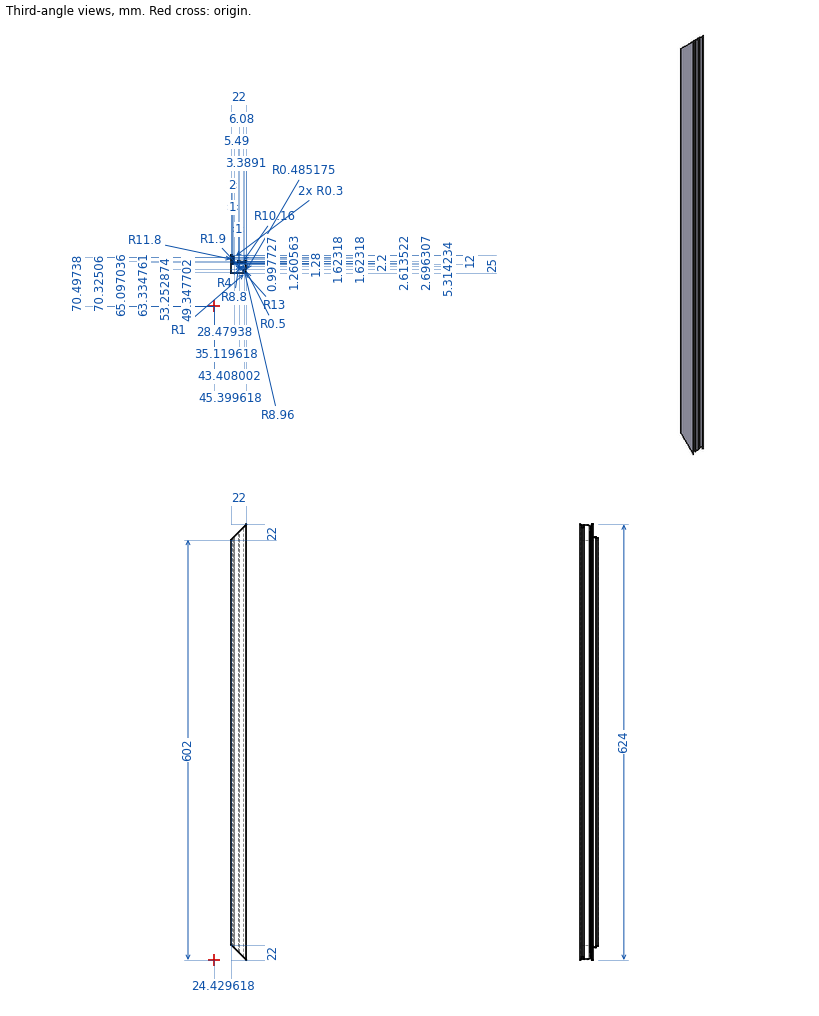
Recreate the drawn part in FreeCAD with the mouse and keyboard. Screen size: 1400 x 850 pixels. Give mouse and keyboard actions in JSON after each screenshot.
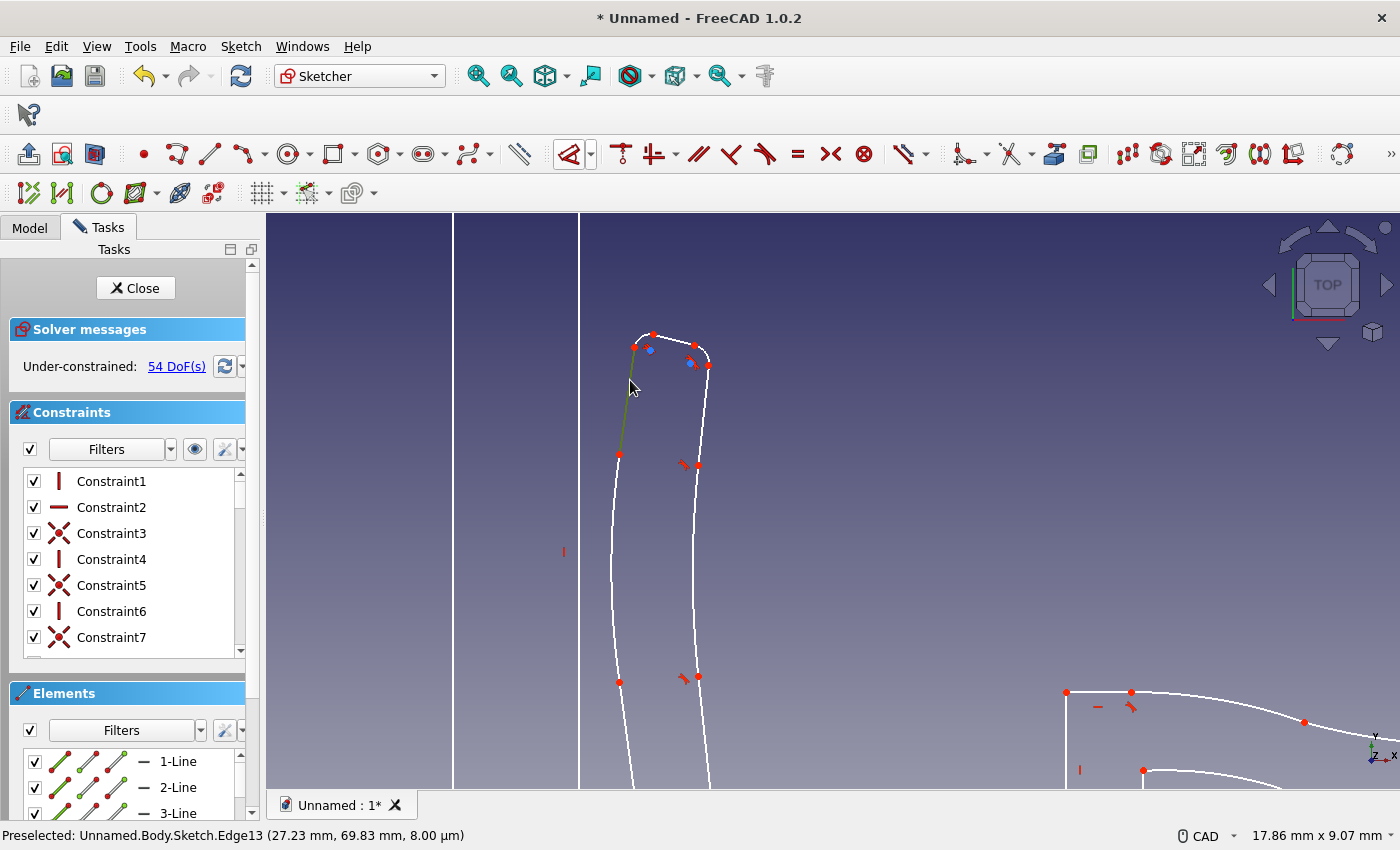
{"action": "left_click", "coordinate": [613, 523]}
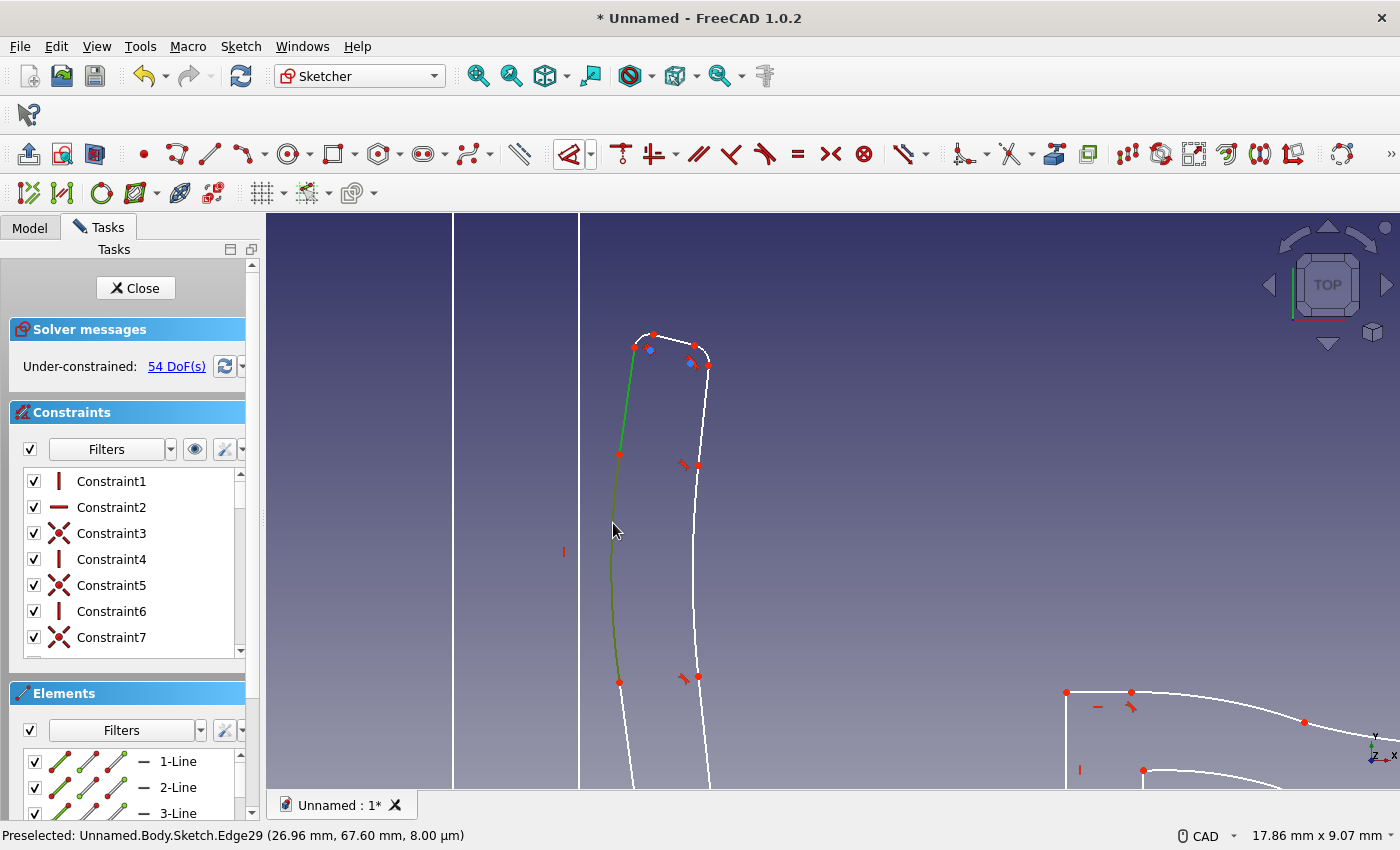
{"action": "key", "text": "t"}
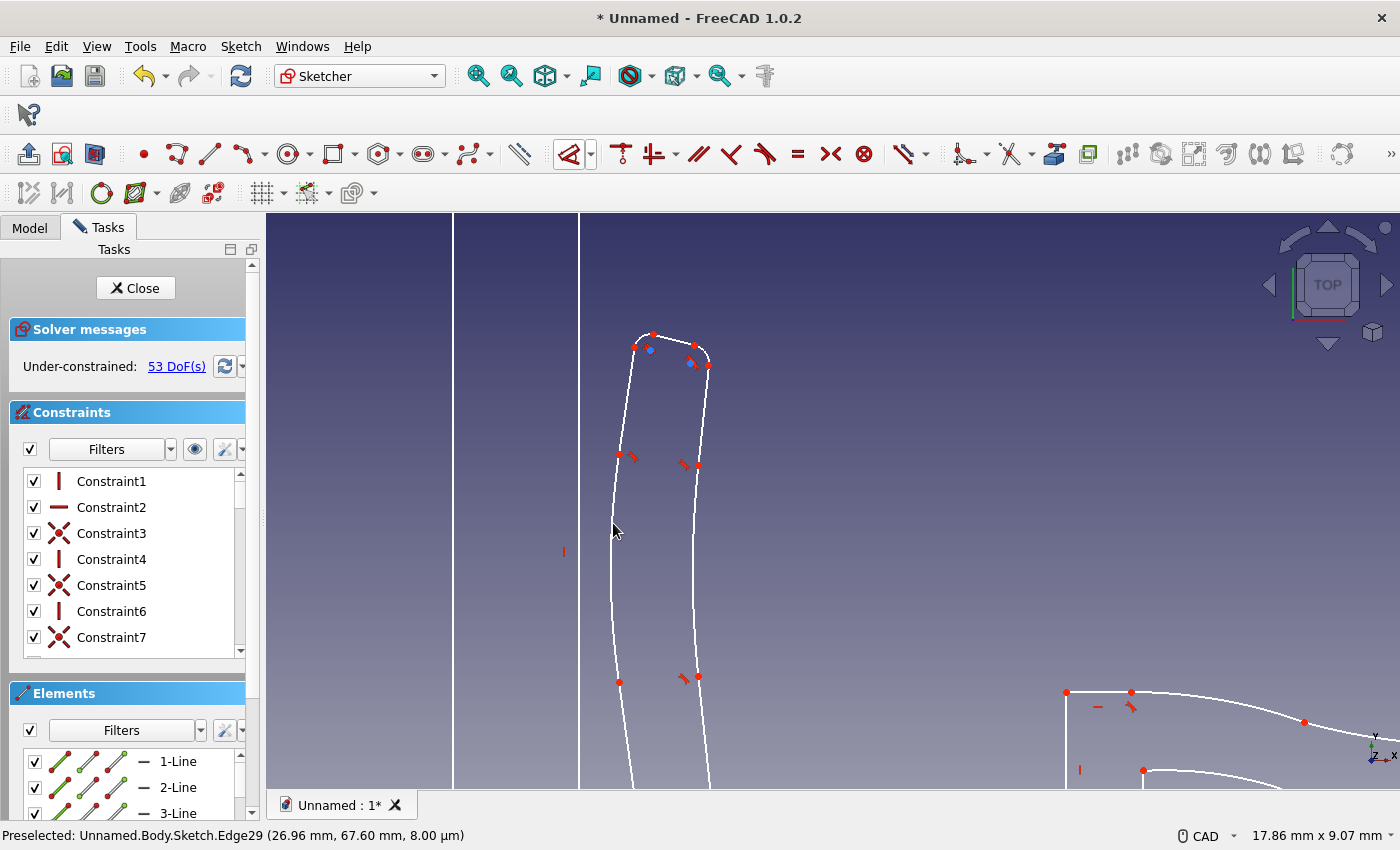
{"action": "scroll", "coordinate": [638, 351], "scroll_direction": "down", "scroll_amount": 7}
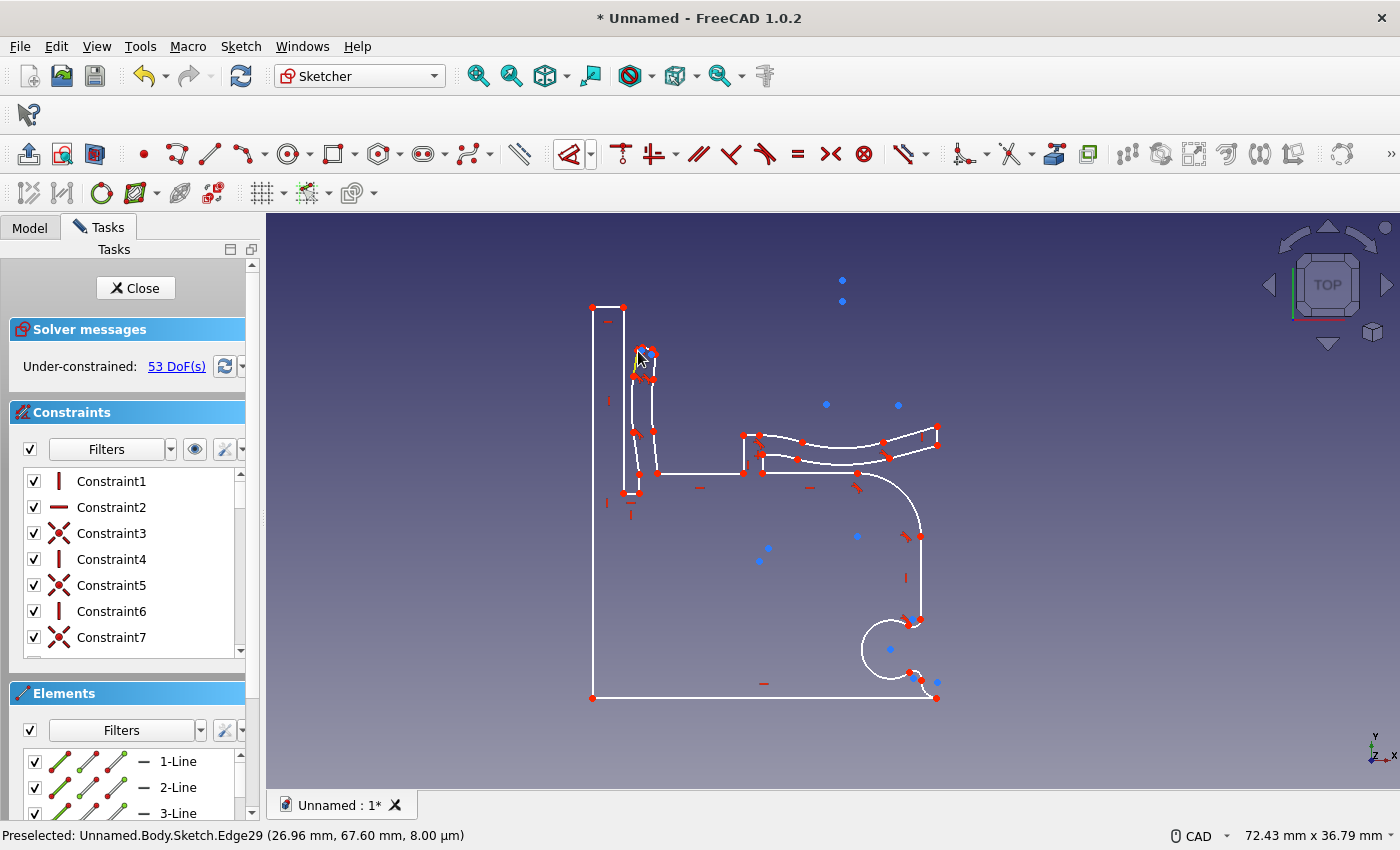
{"action": "left_click", "coordinate": [635, 445]}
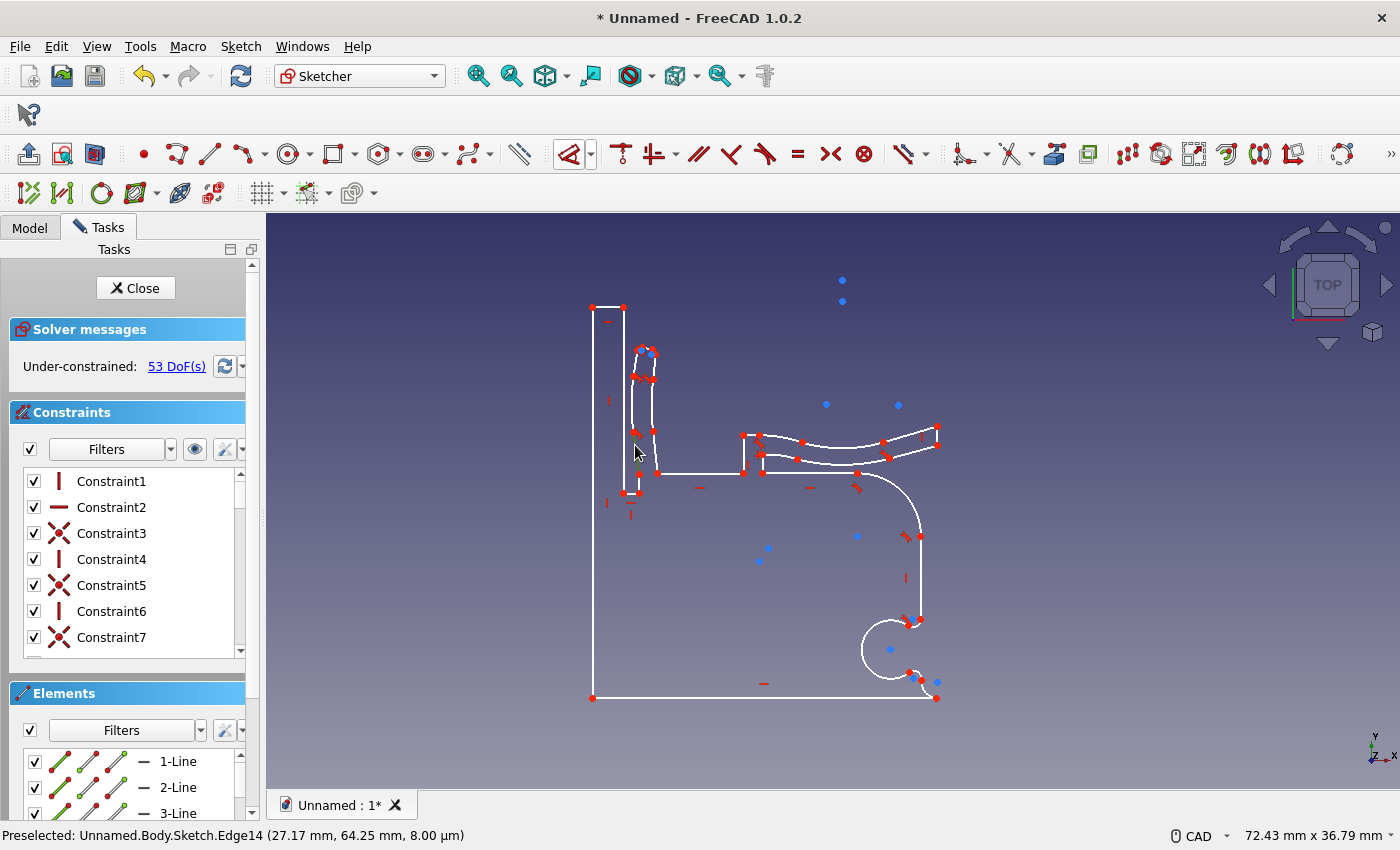
{"action": "scroll", "coordinate": [632, 422], "scroll_direction": "up", "scroll_amount": 3}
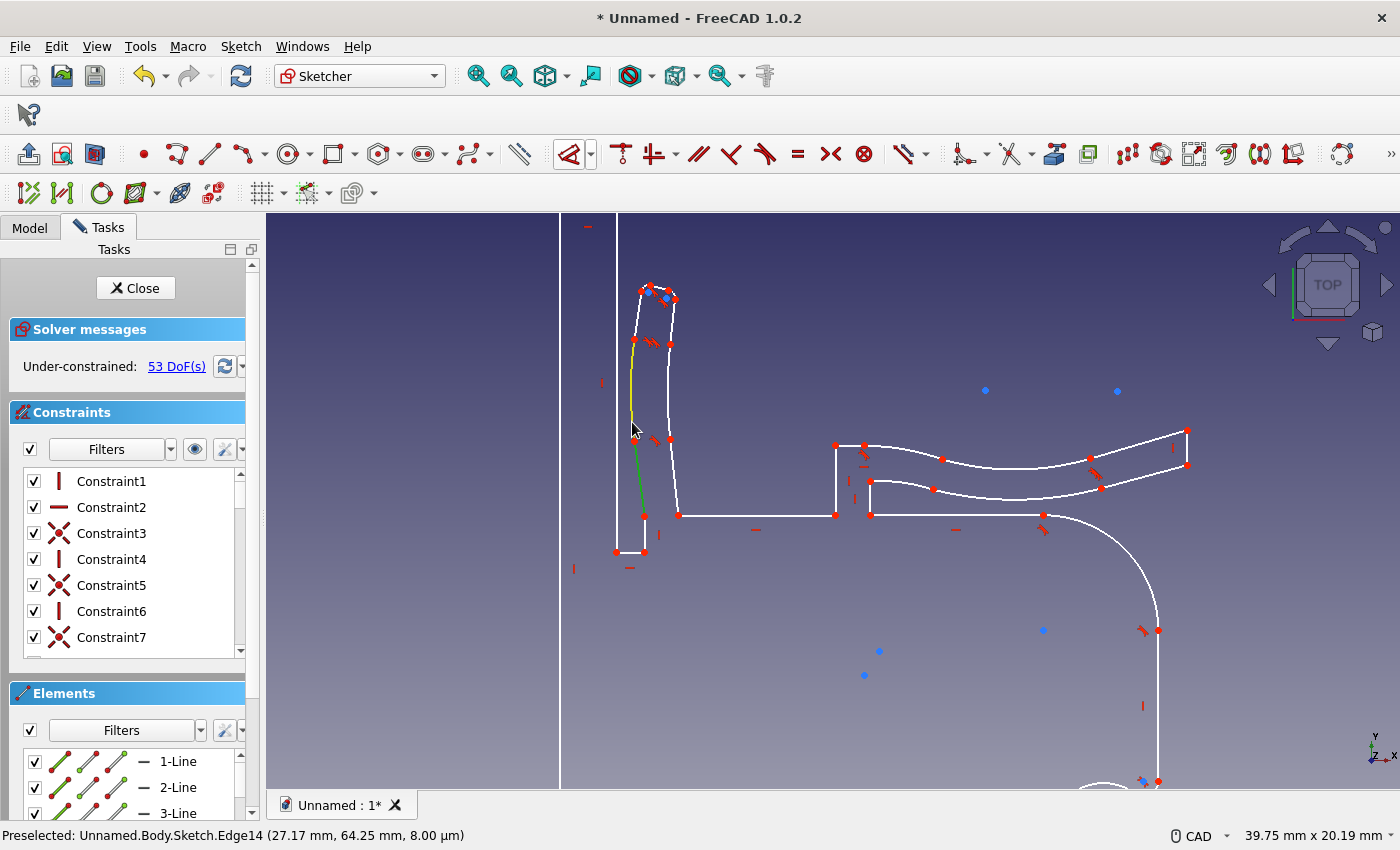
{"action": "left_click", "coordinate": [632, 421]}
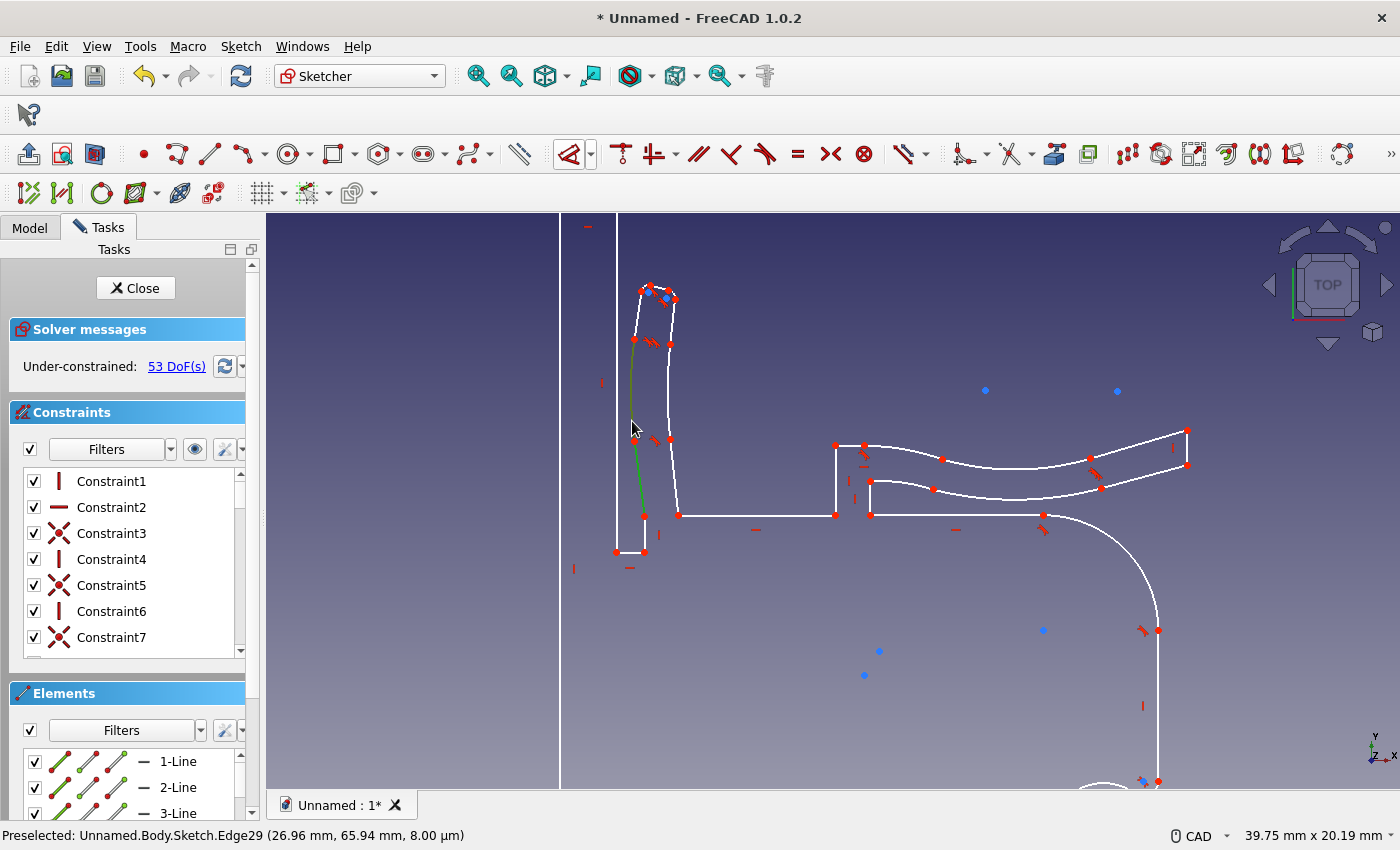
{"action": "left_click", "coordinate": [765, 154]}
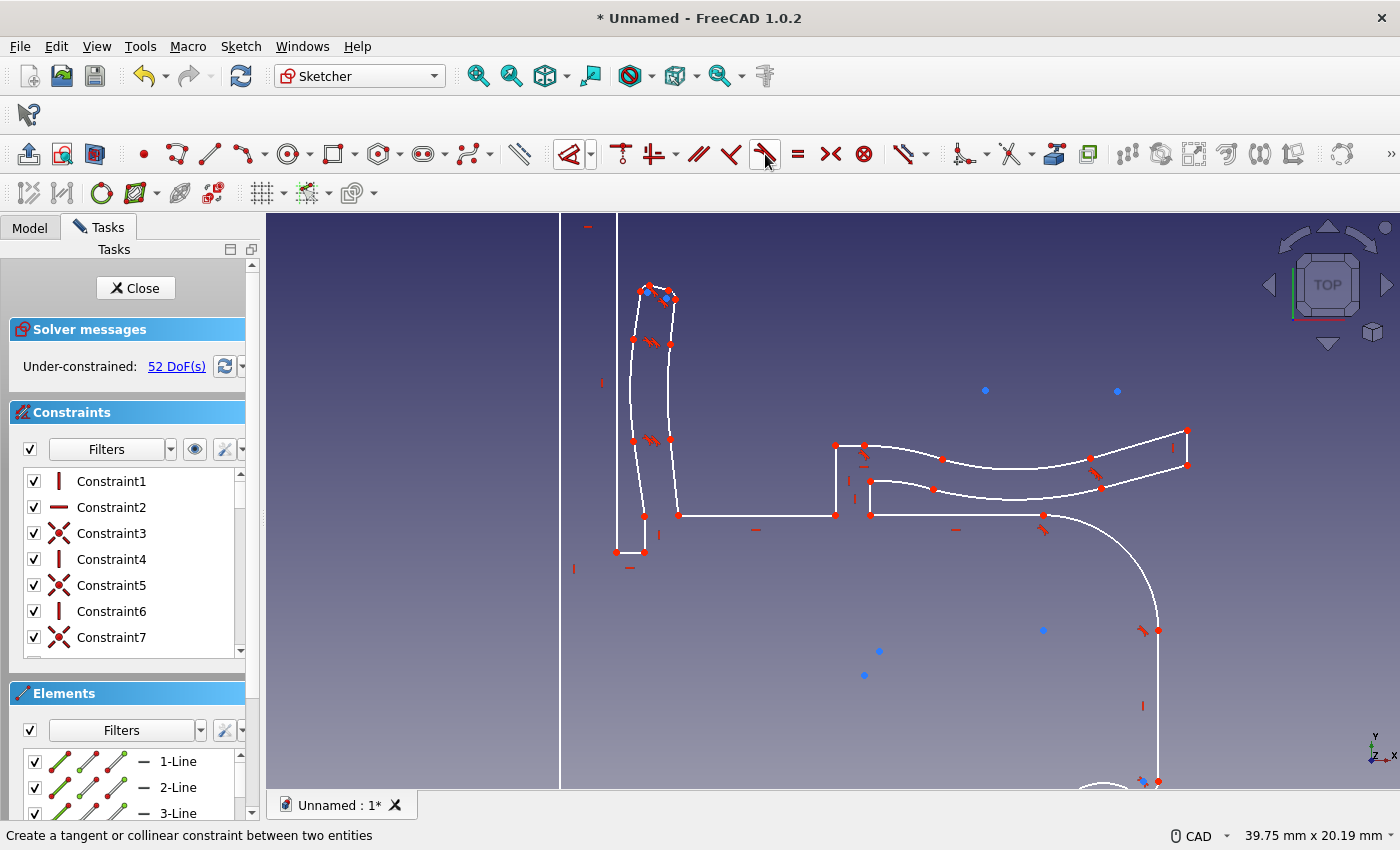
{"action": "scroll", "coordinate": [632, 421], "scroll_direction": "down", "scroll_amount": 3}